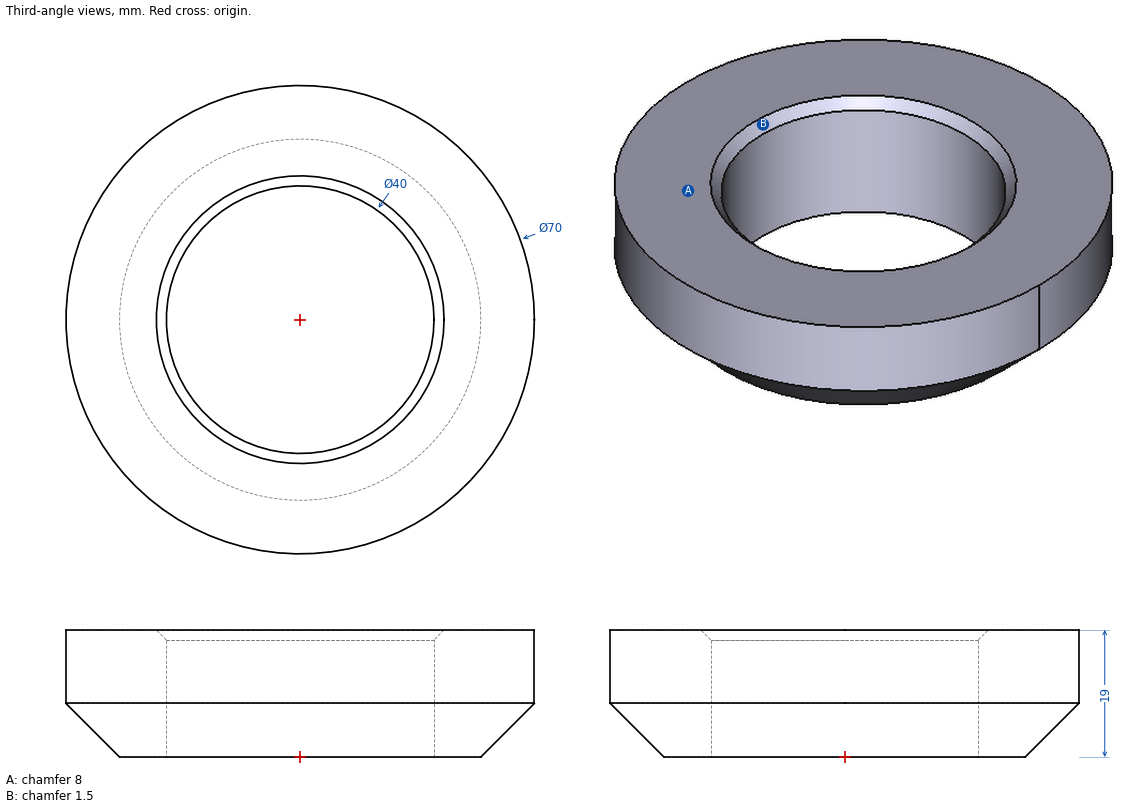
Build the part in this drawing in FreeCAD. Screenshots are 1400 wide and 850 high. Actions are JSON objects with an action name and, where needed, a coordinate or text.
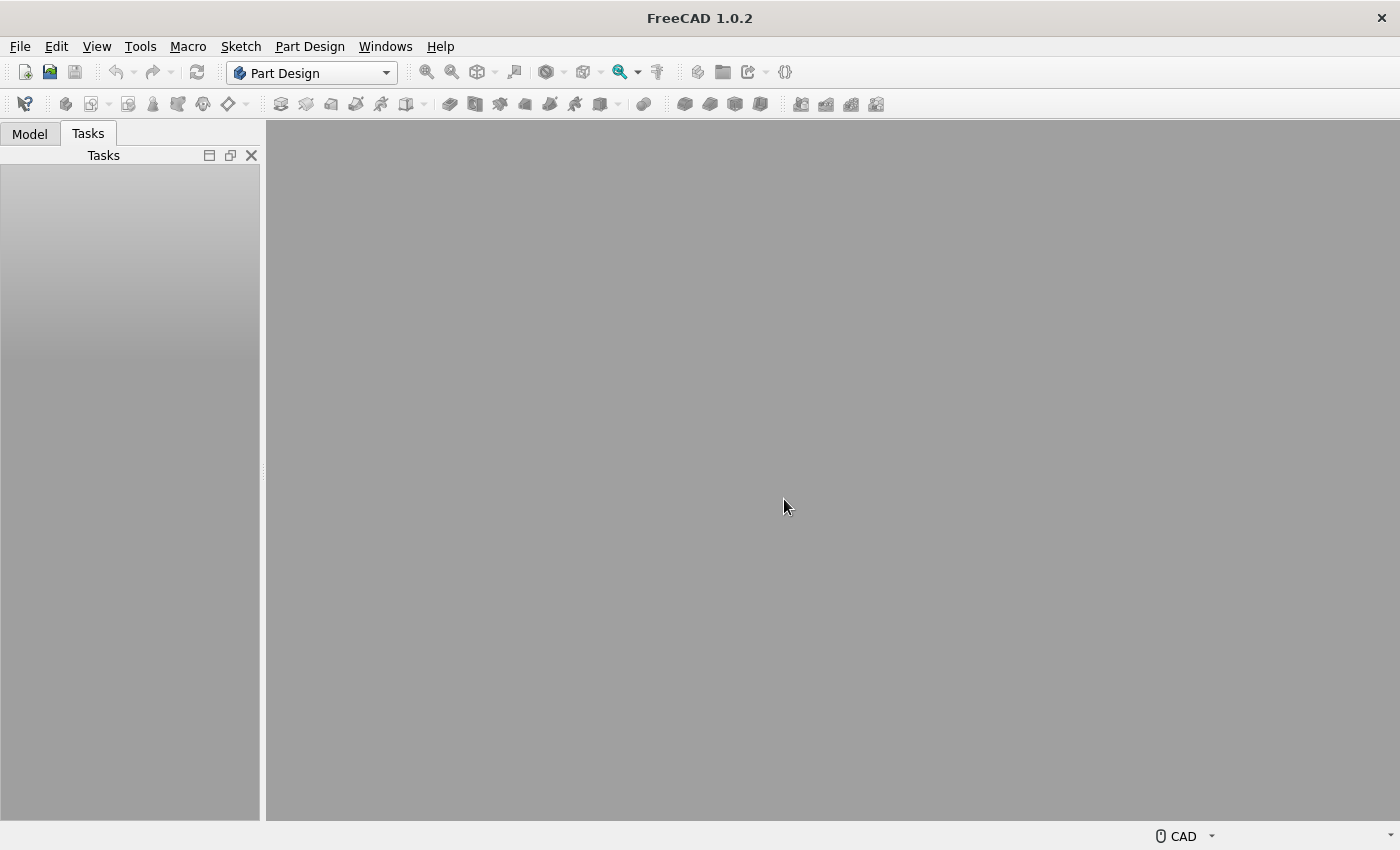
{"action": "key", "text": "ctrl+n"}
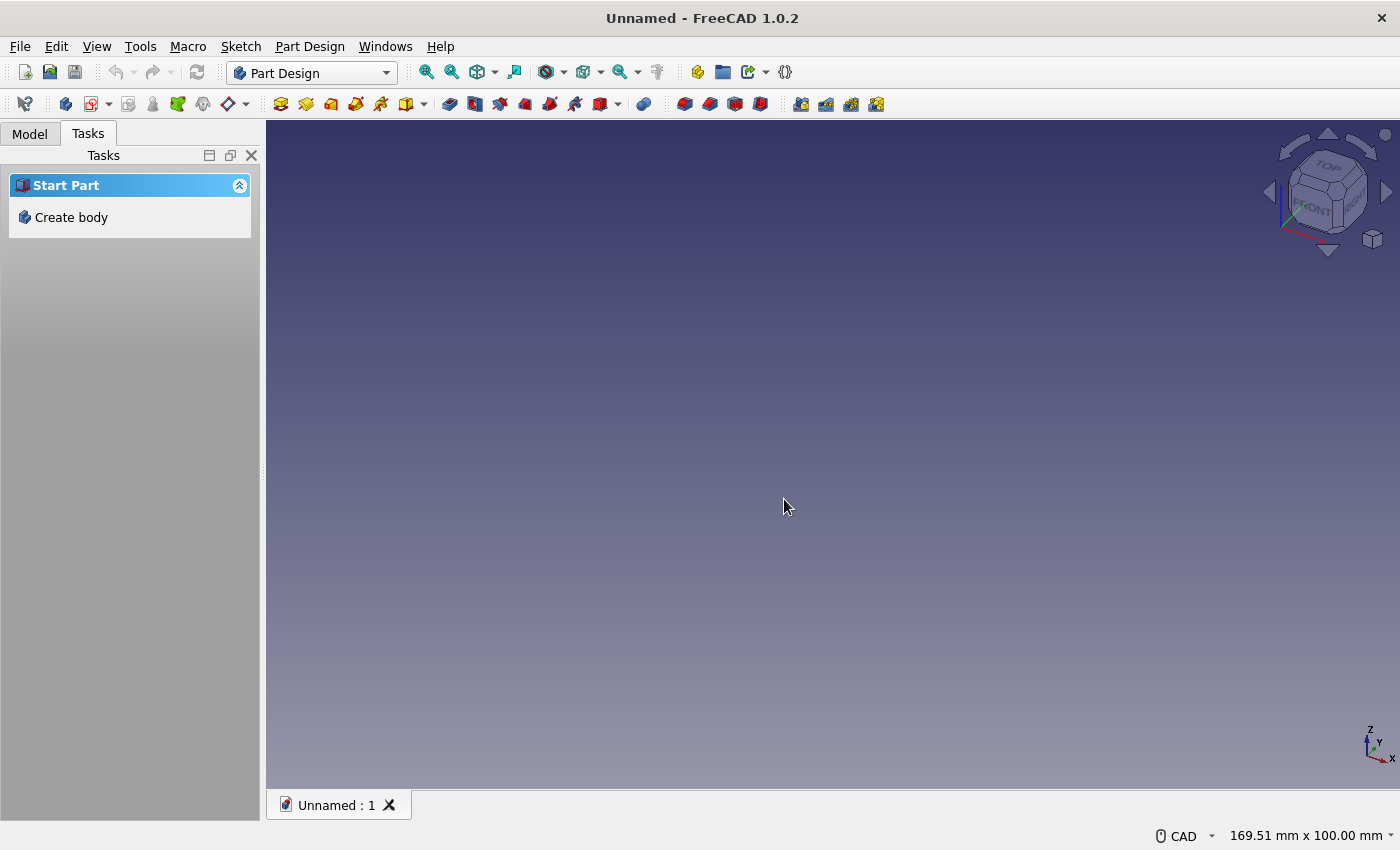
{"action": "left_click", "coordinate": [90, 104]}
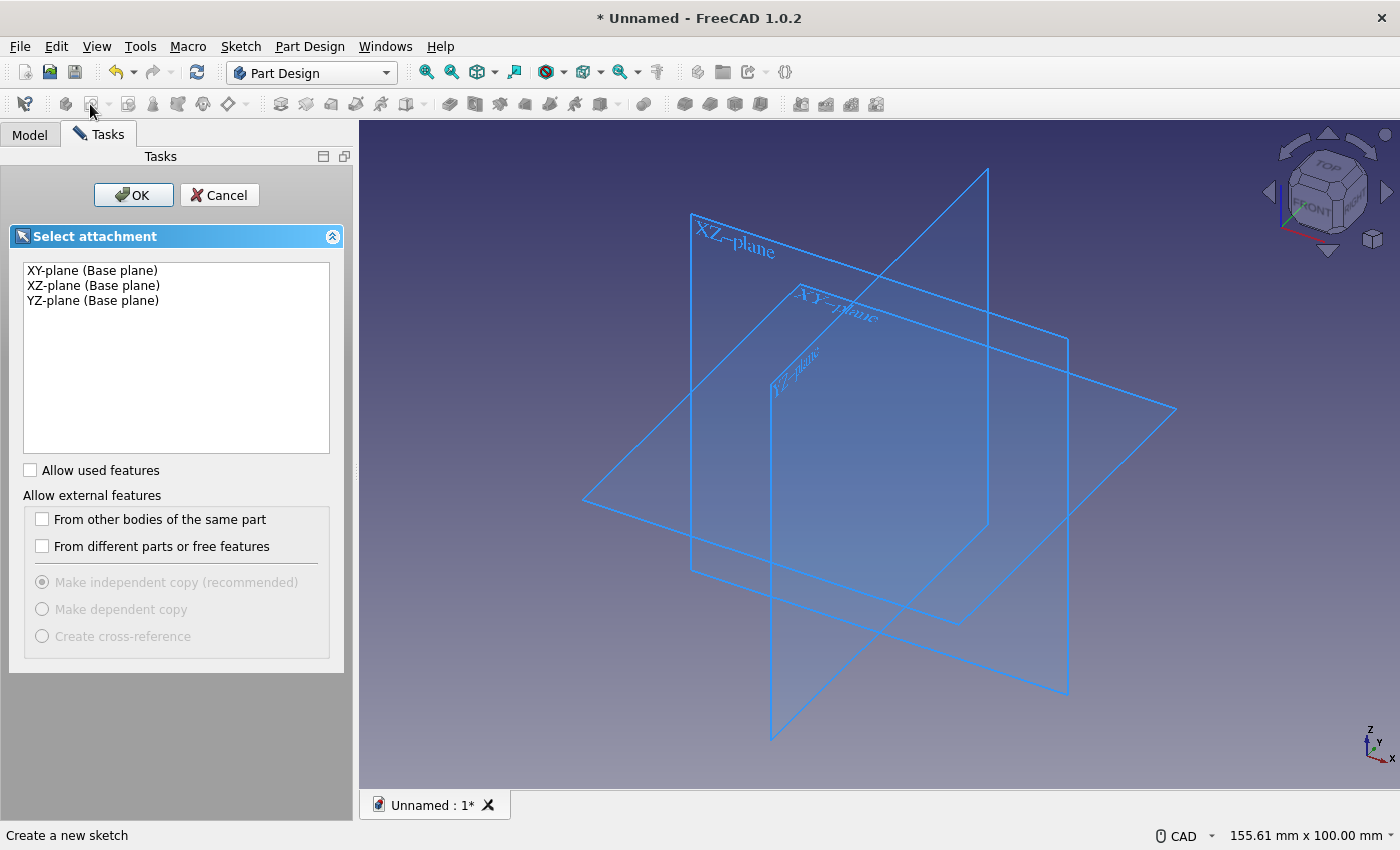
{"action": "left_click", "coordinate": [84, 270]}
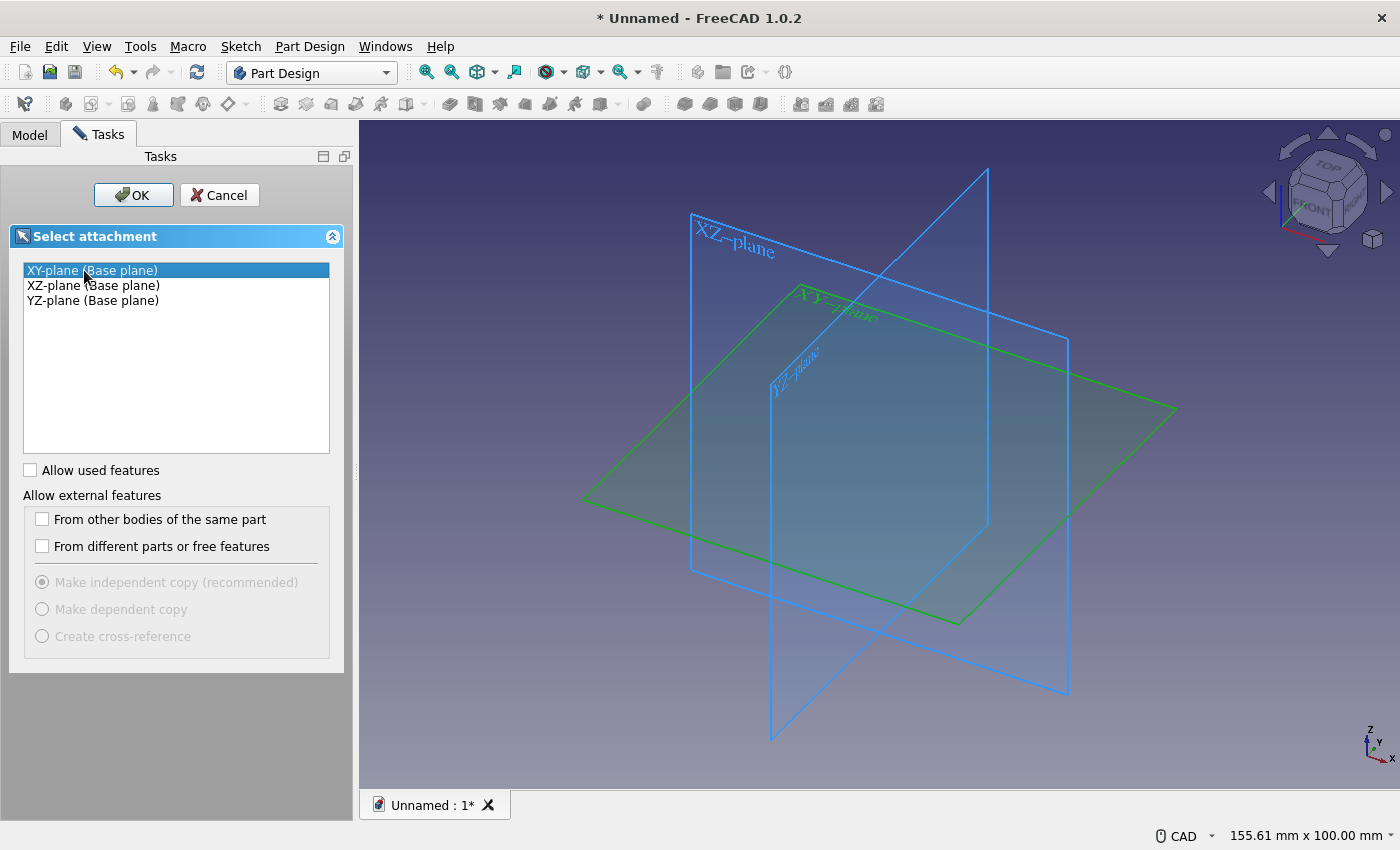
{"action": "left_click", "coordinate": [134, 195]}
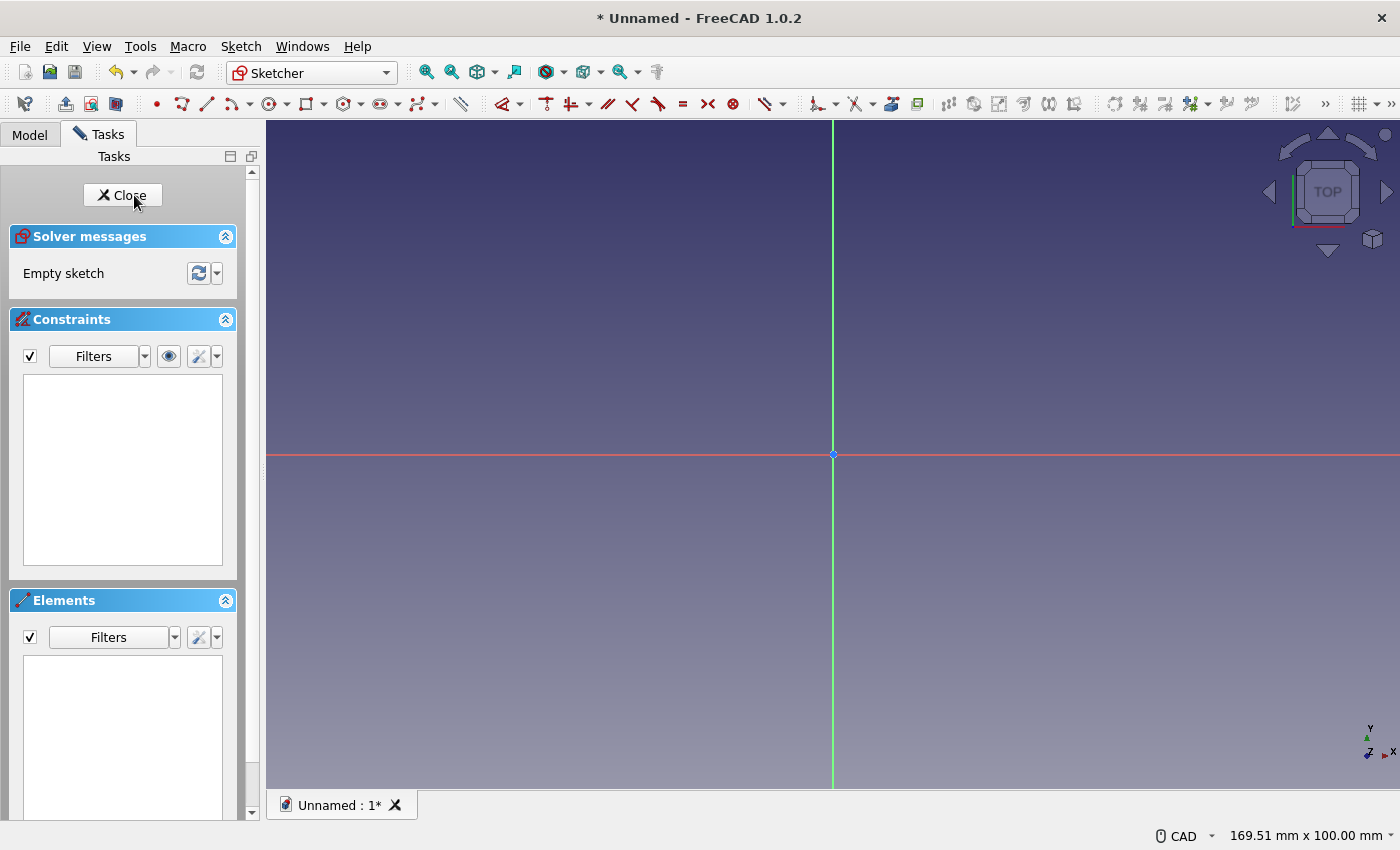
{"action": "left_click", "coordinate": [268, 104]}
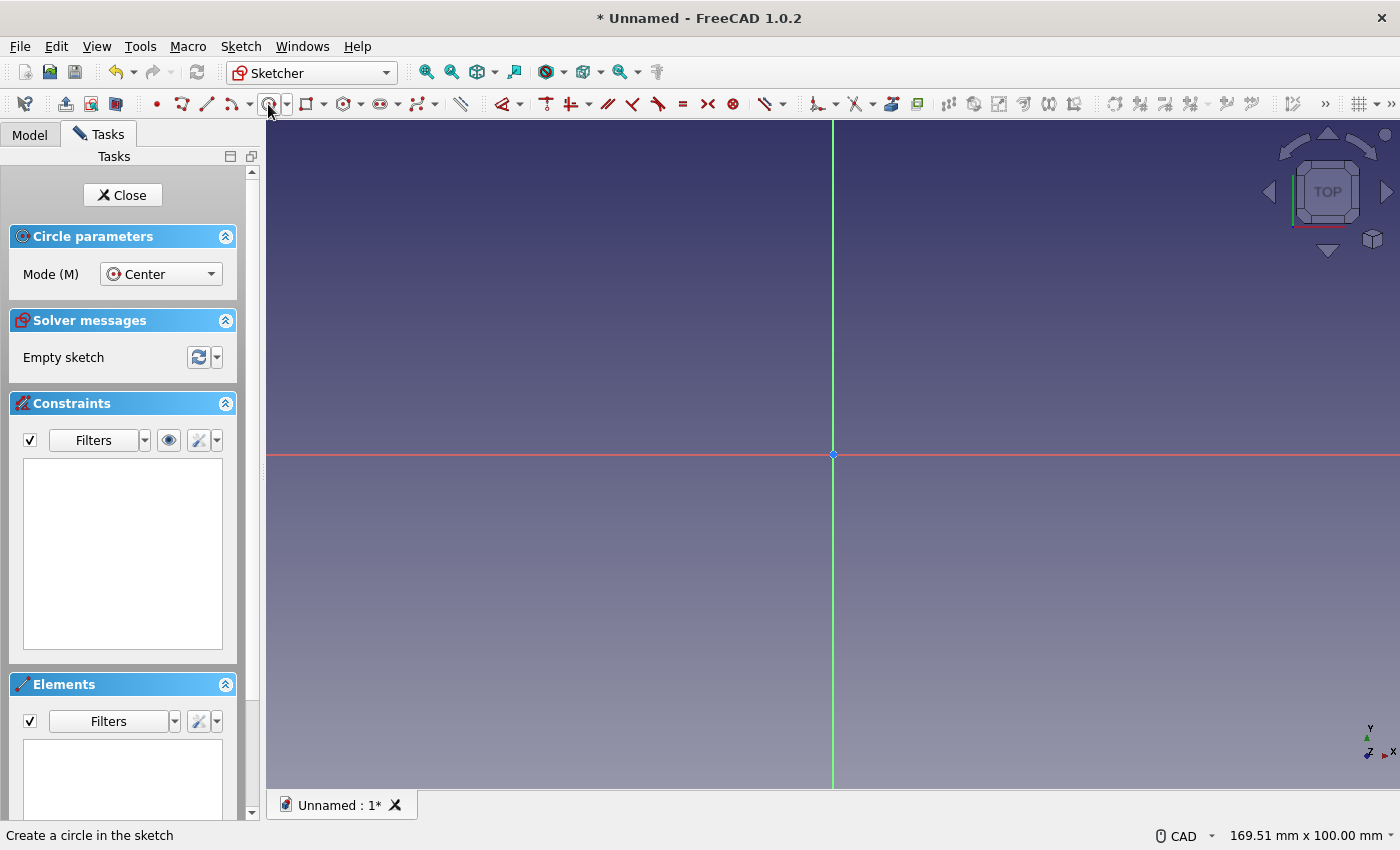
{"action": "left_click", "coordinate": [833, 454]}
{"action": "mouse_move", "coordinate": [999, 289]}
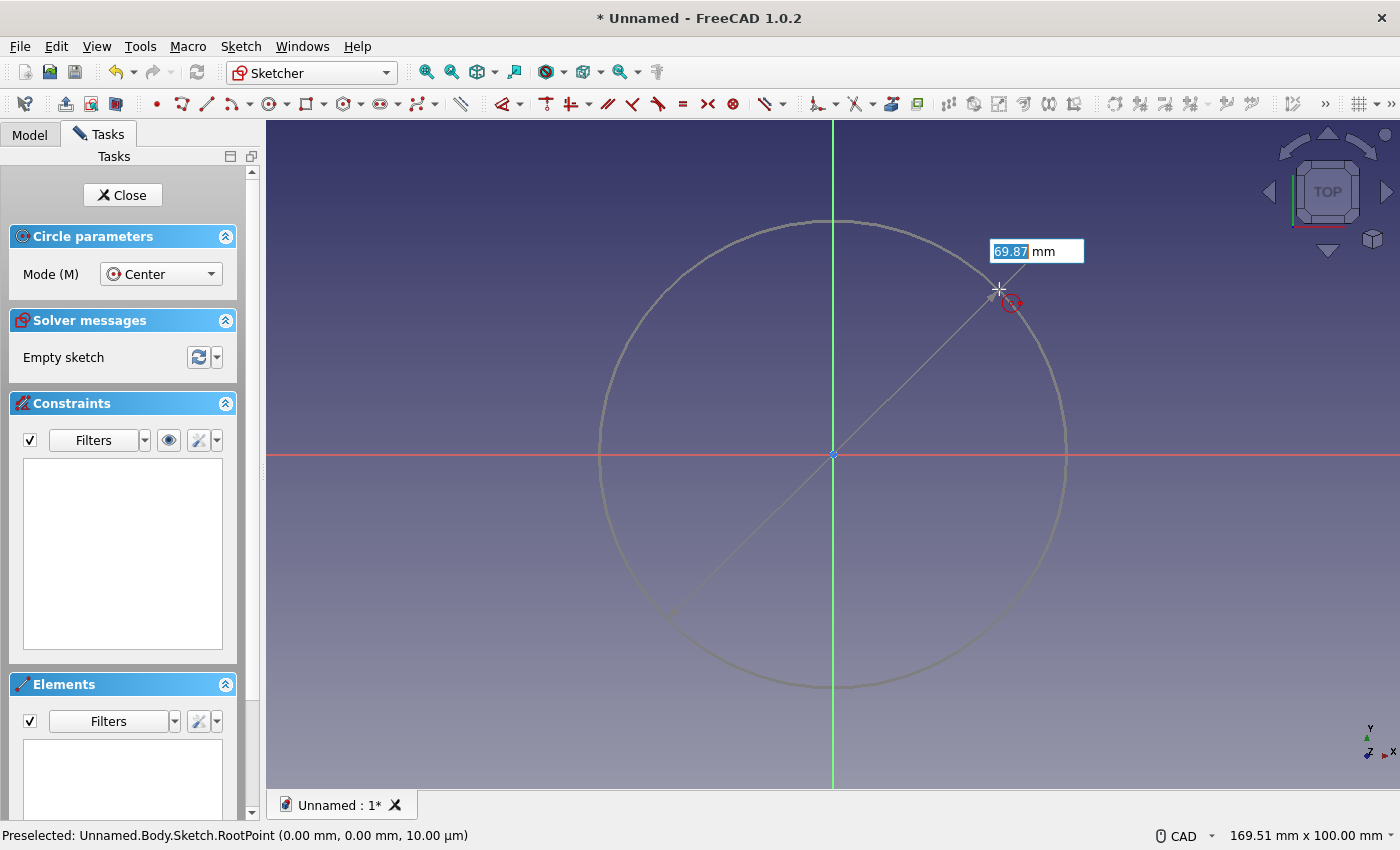
{"action": "type", "text": "70"}
{"action": "key", "text": "Return"}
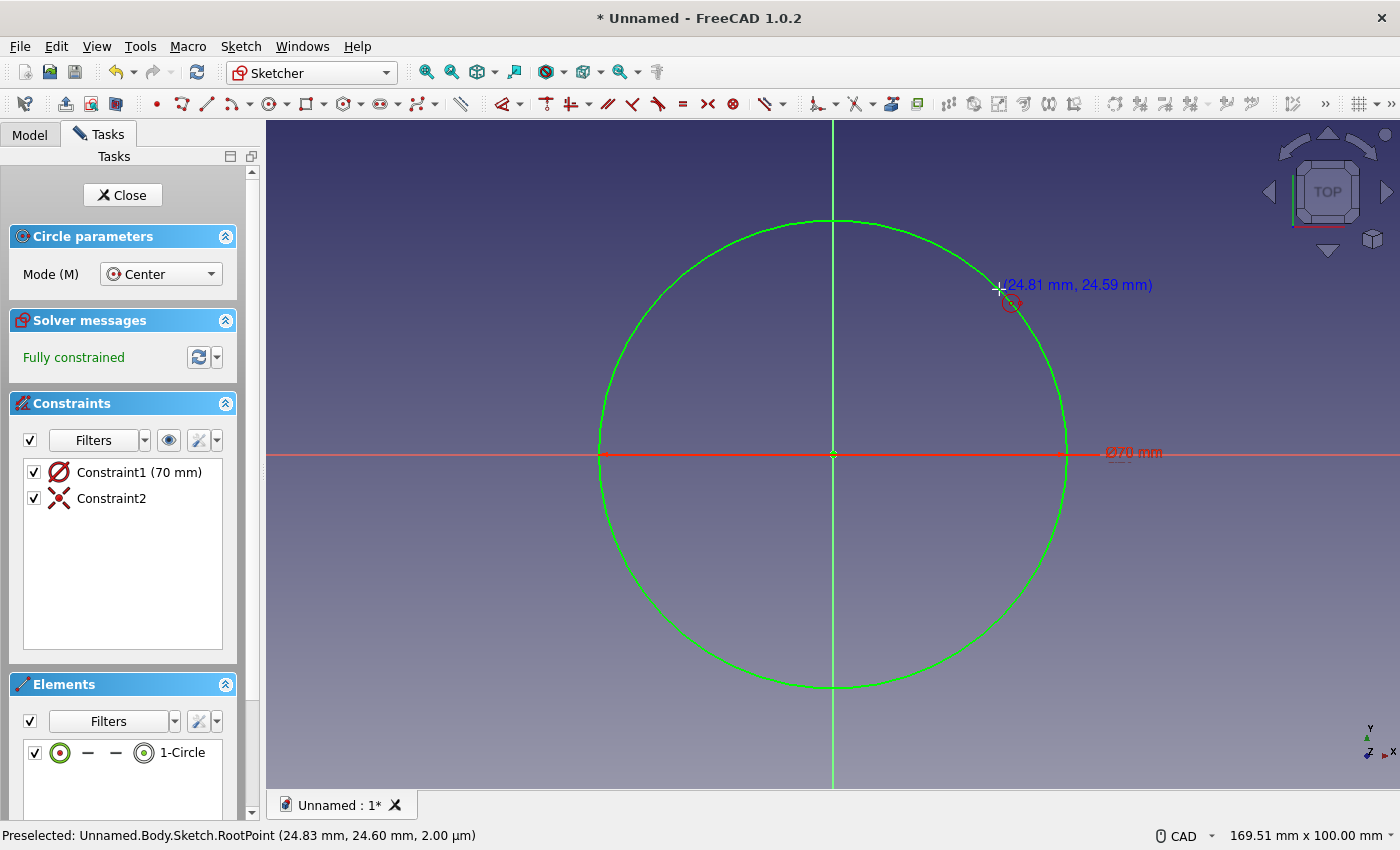
{"action": "left_click", "coordinate": [833, 454]}
{"action": "mouse_move", "coordinate": [928, 360]}